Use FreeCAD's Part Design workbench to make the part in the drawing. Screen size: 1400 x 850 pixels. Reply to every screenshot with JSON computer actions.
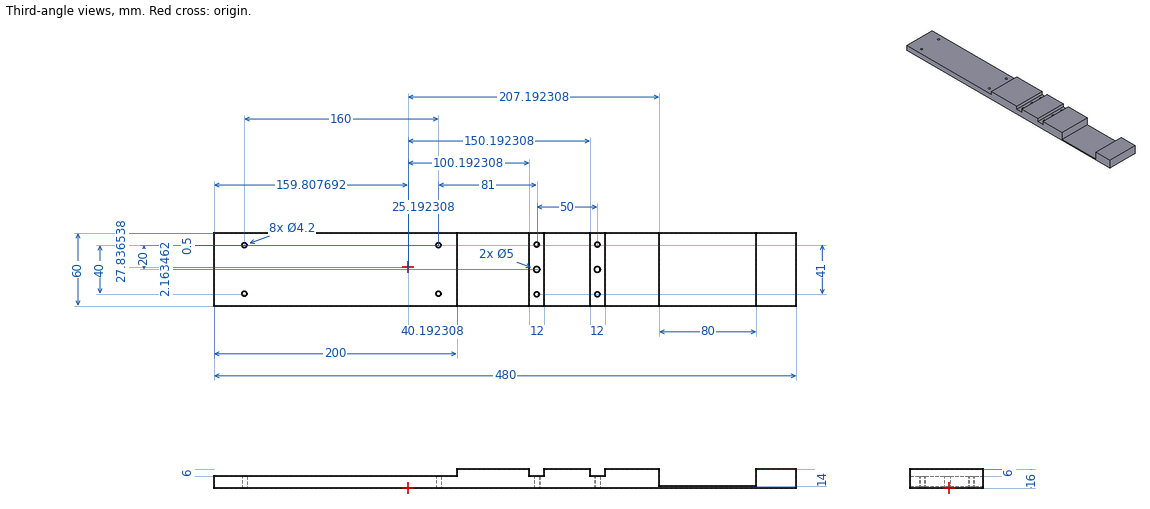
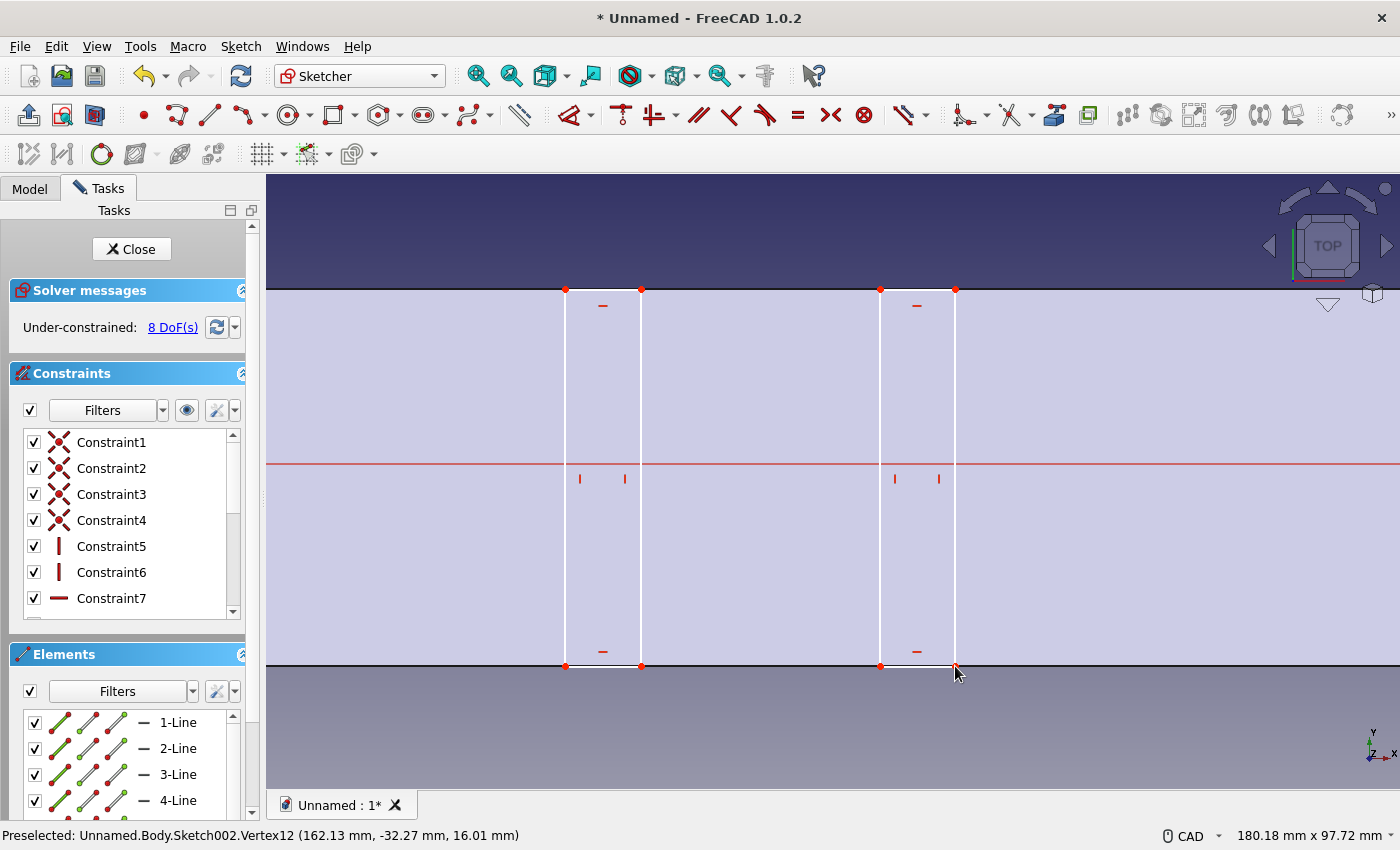
{"action": "left_click", "coordinate": [568, 116]}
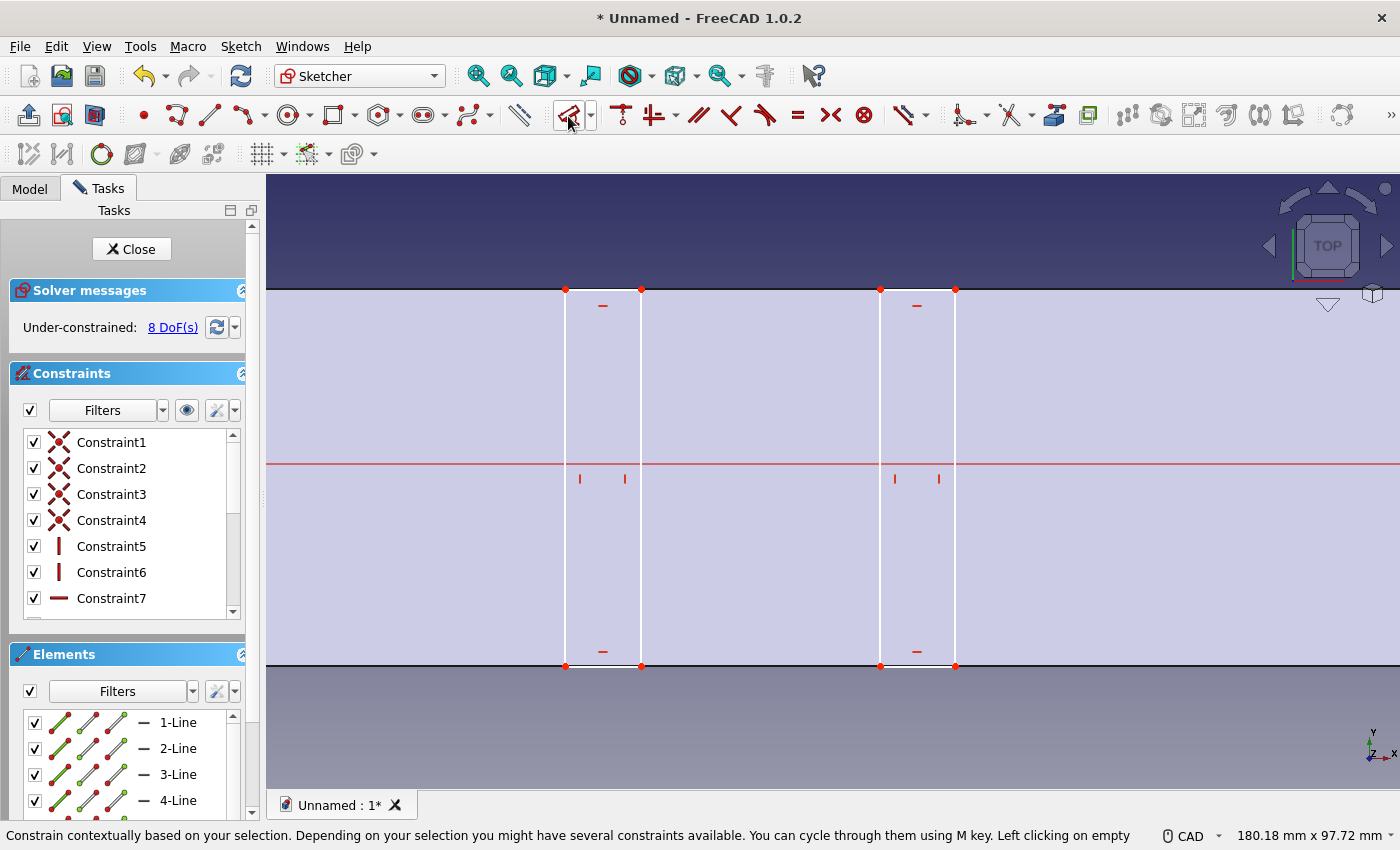
{"action": "left_click", "coordinate": [565, 403]}
{"action": "left_click", "coordinate": [531, 478]}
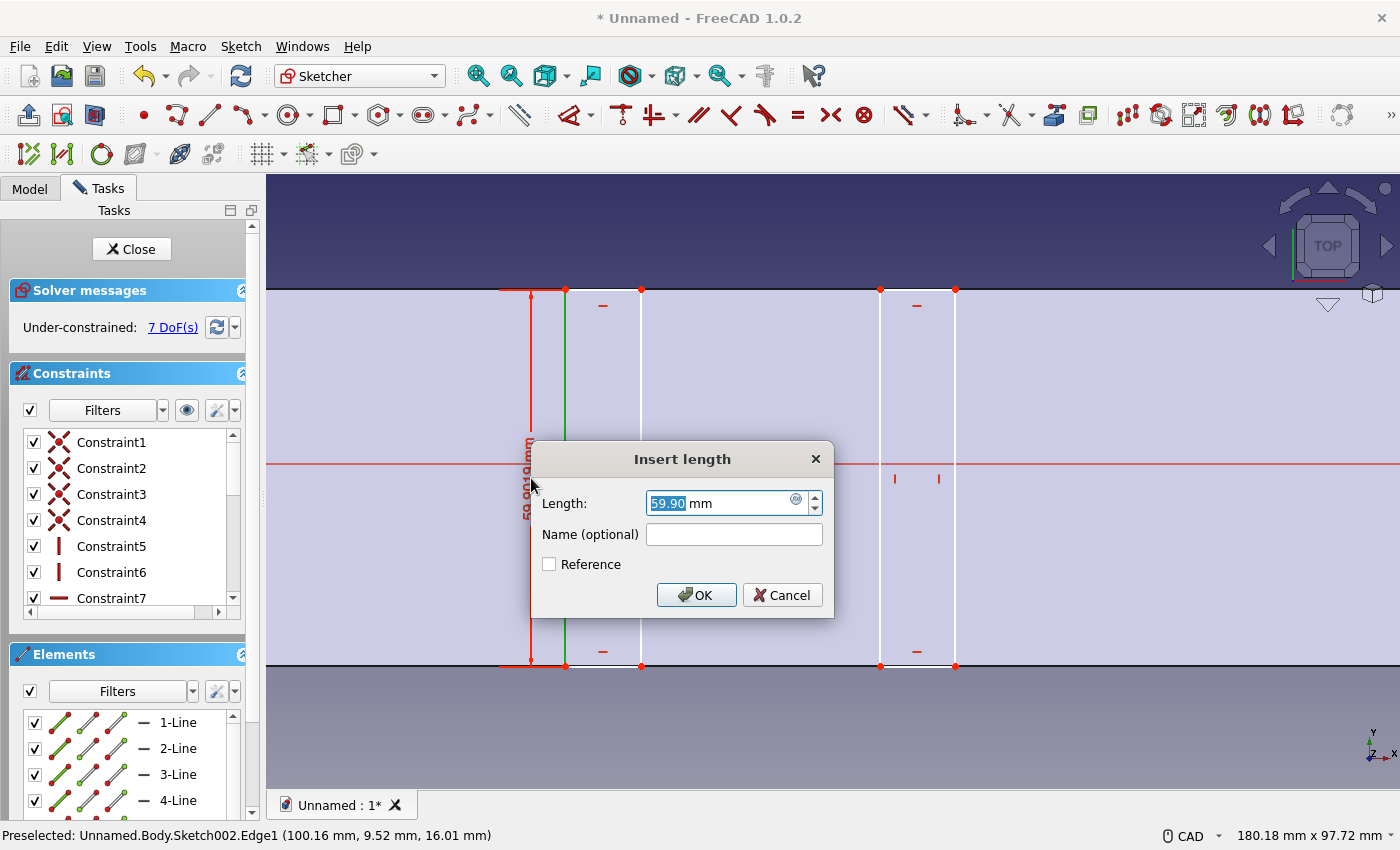
{"action": "type", "text": "60"}
{"action": "key", "text": "Return"}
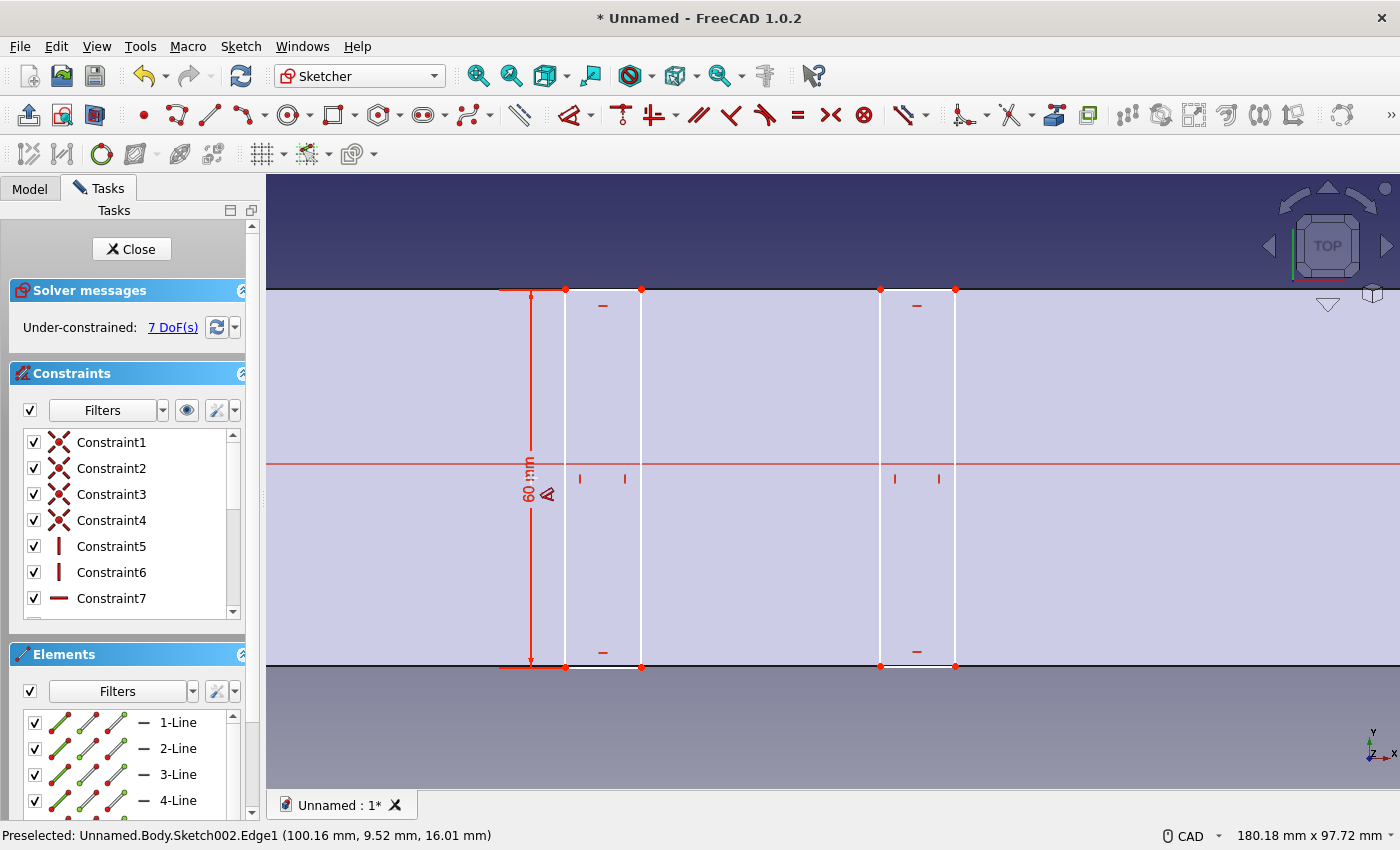
{"action": "left_click", "coordinate": [588, 668]}
{"action": "left_click", "coordinate": [603, 702]}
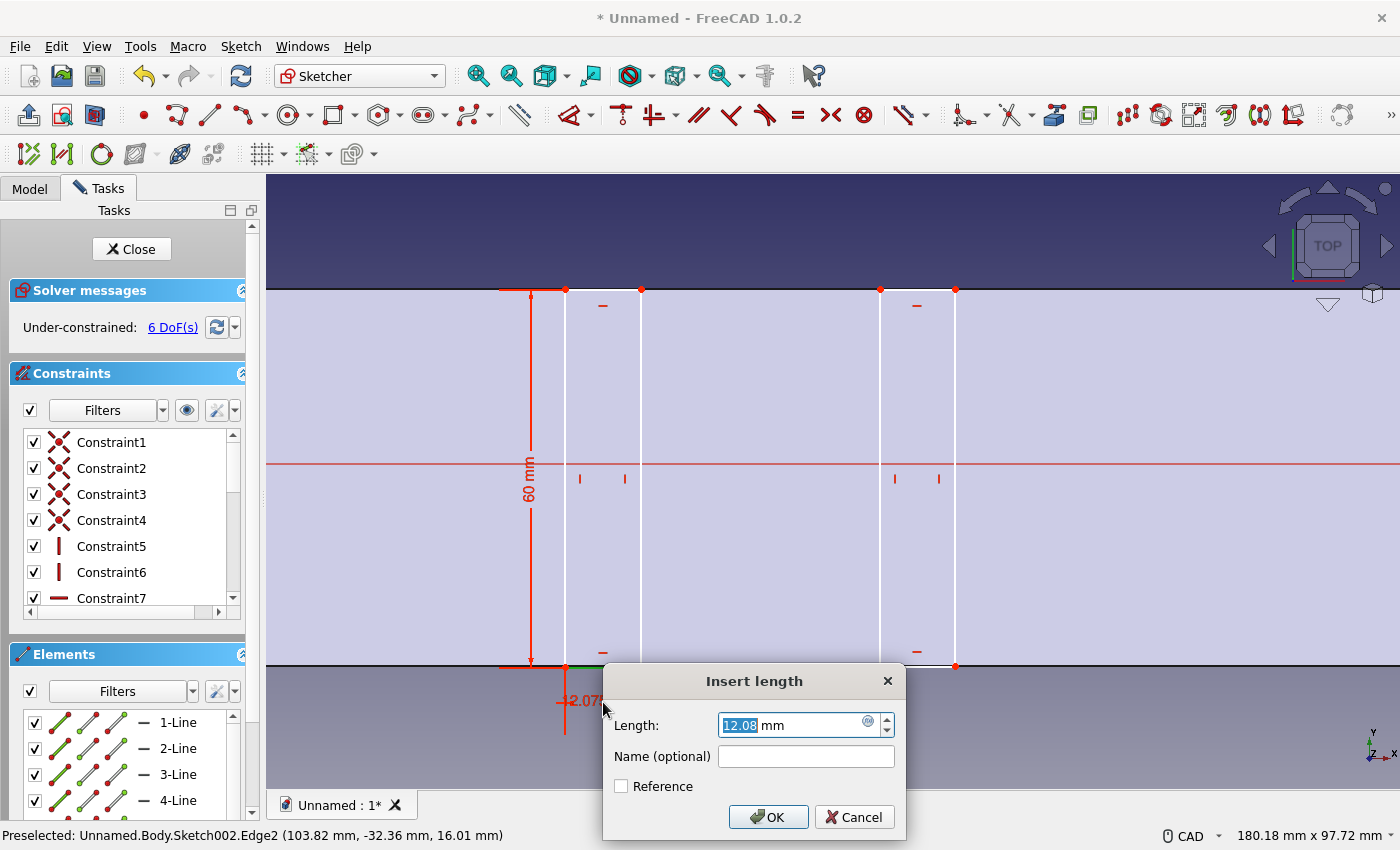
{"action": "type", "text": "12"}
{"action": "key", "text": "Return"}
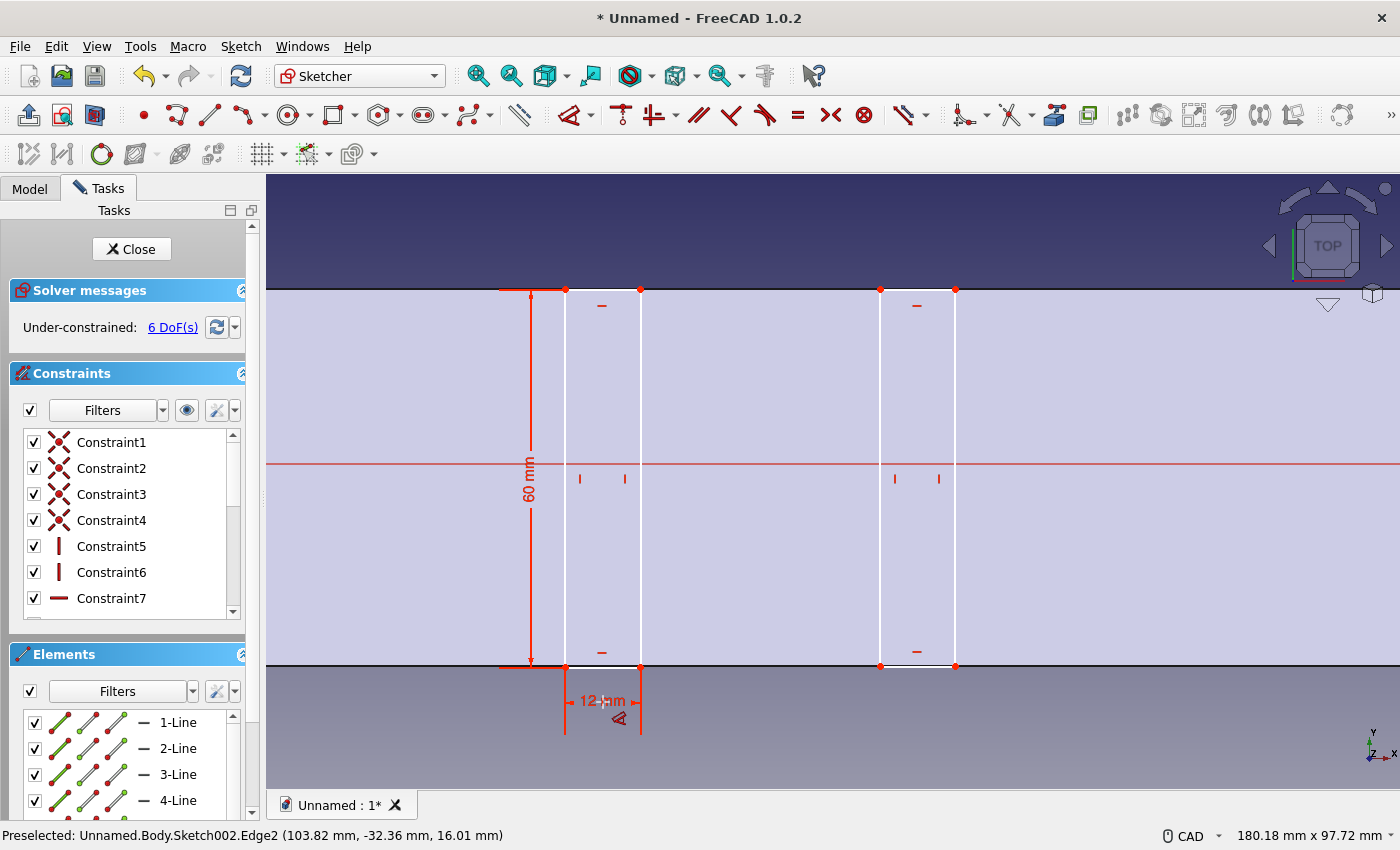
{"action": "left_click", "coordinate": [880, 403]}
{"action": "left_click", "coordinate": [914, 478]}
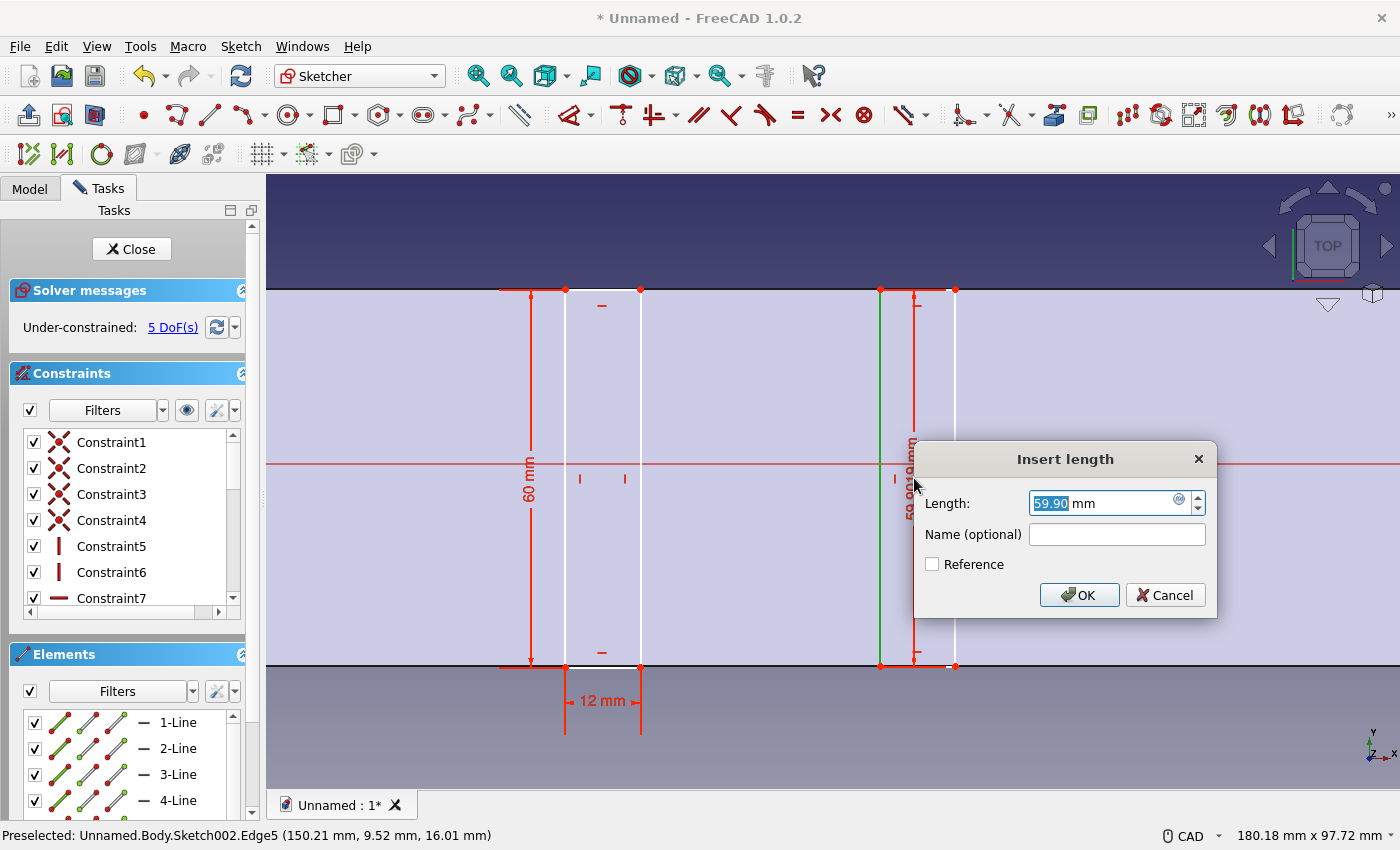
{"action": "type", "text": "60"}
{"action": "key", "text": "Return"}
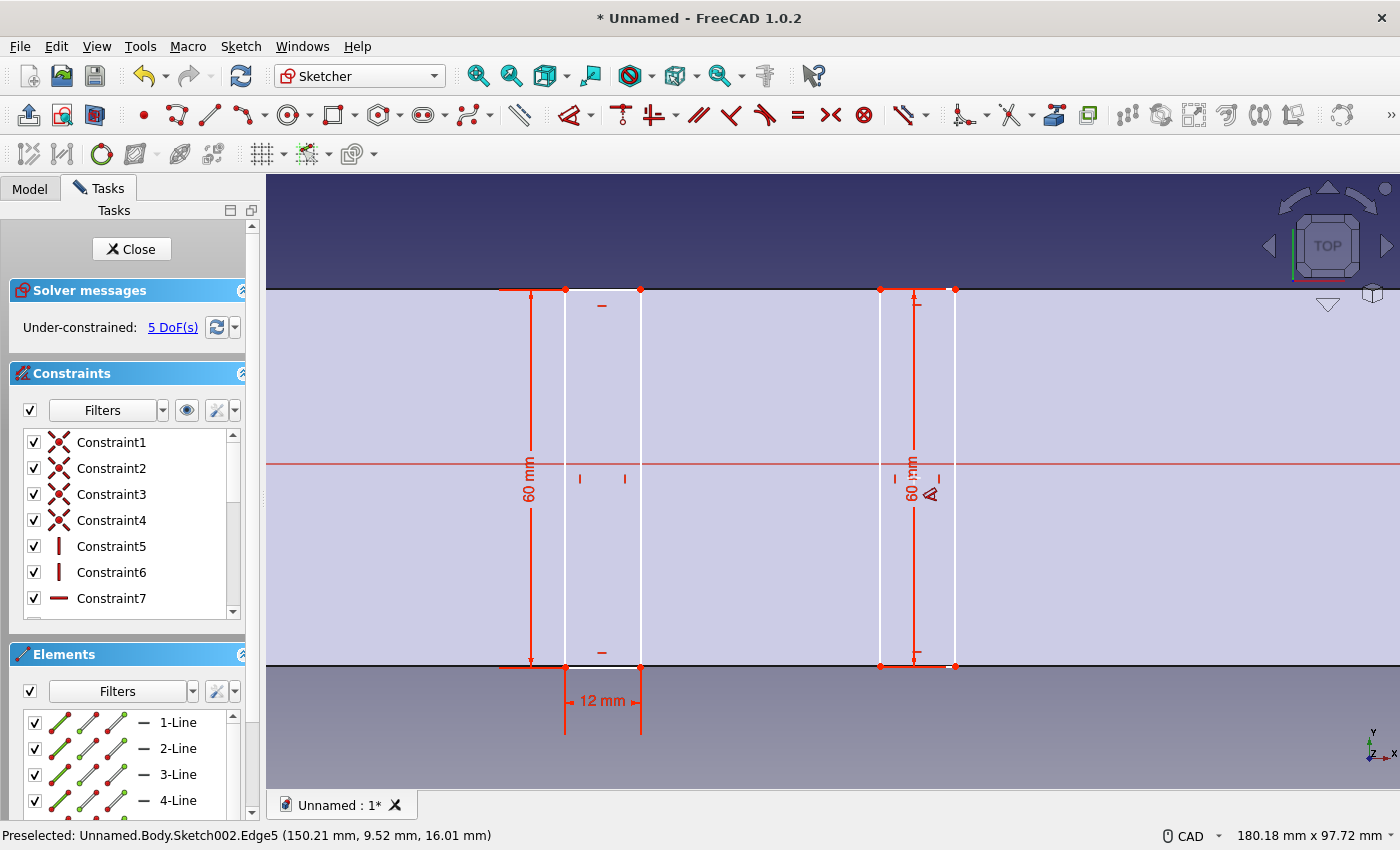
{"action": "left_click", "coordinate": [903, 667]}
{"action": "left_click", "coordinate": [918, 701]}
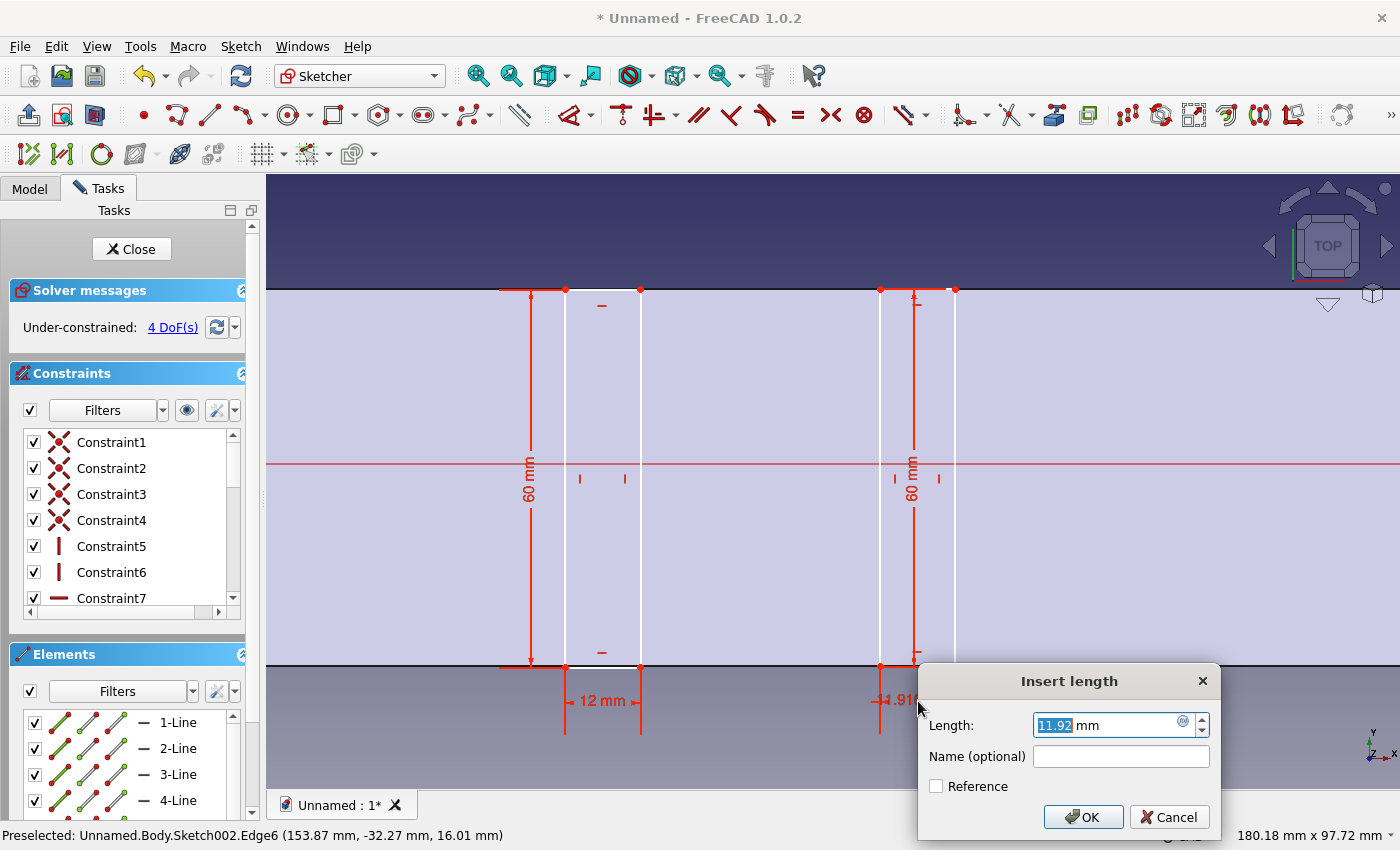
{"action": "type", "text": "12"}
{"action": "key", "text": "Return"}